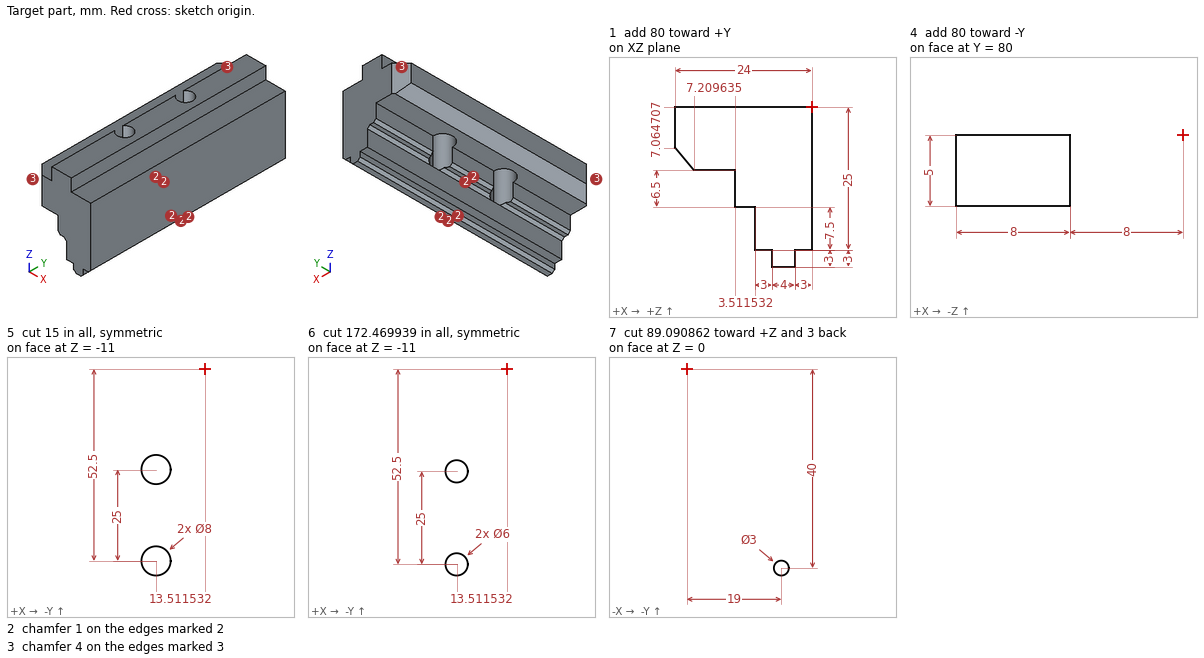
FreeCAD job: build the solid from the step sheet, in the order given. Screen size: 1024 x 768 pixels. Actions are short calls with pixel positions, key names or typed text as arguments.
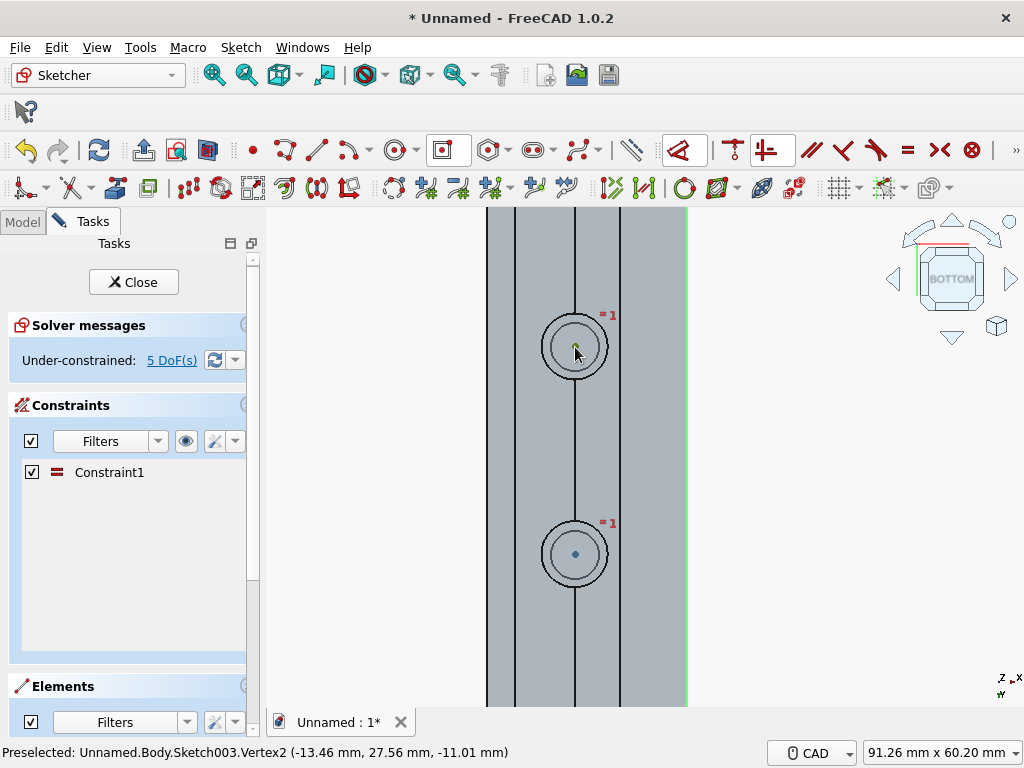
click(790, 150)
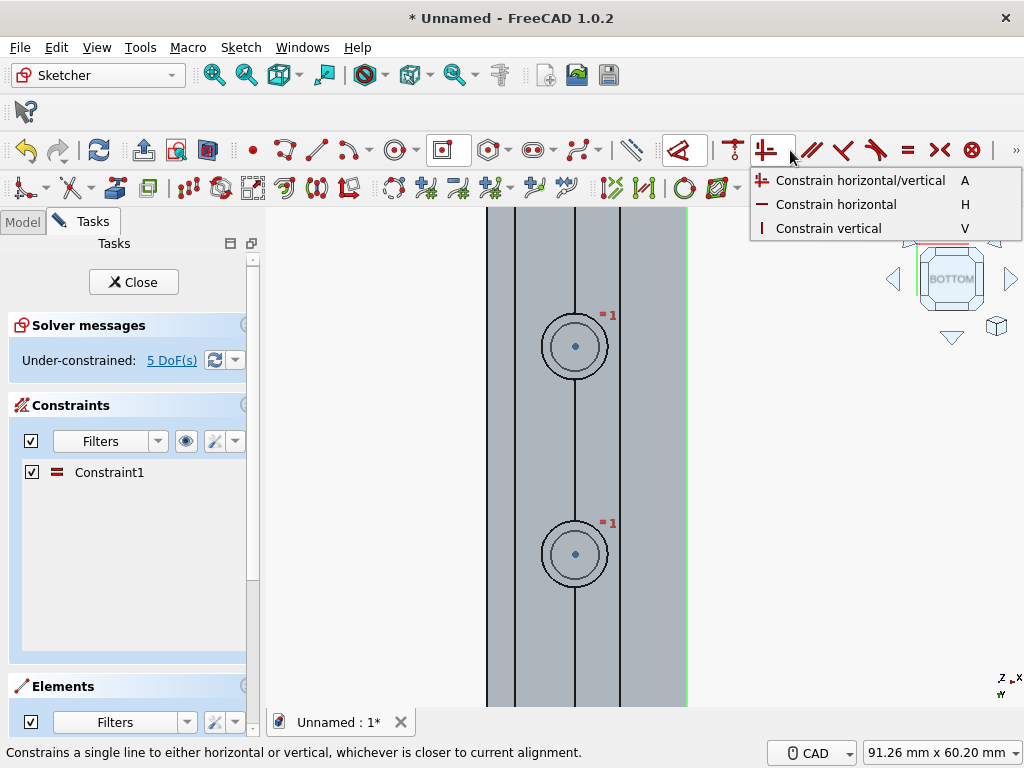
click(886, 228)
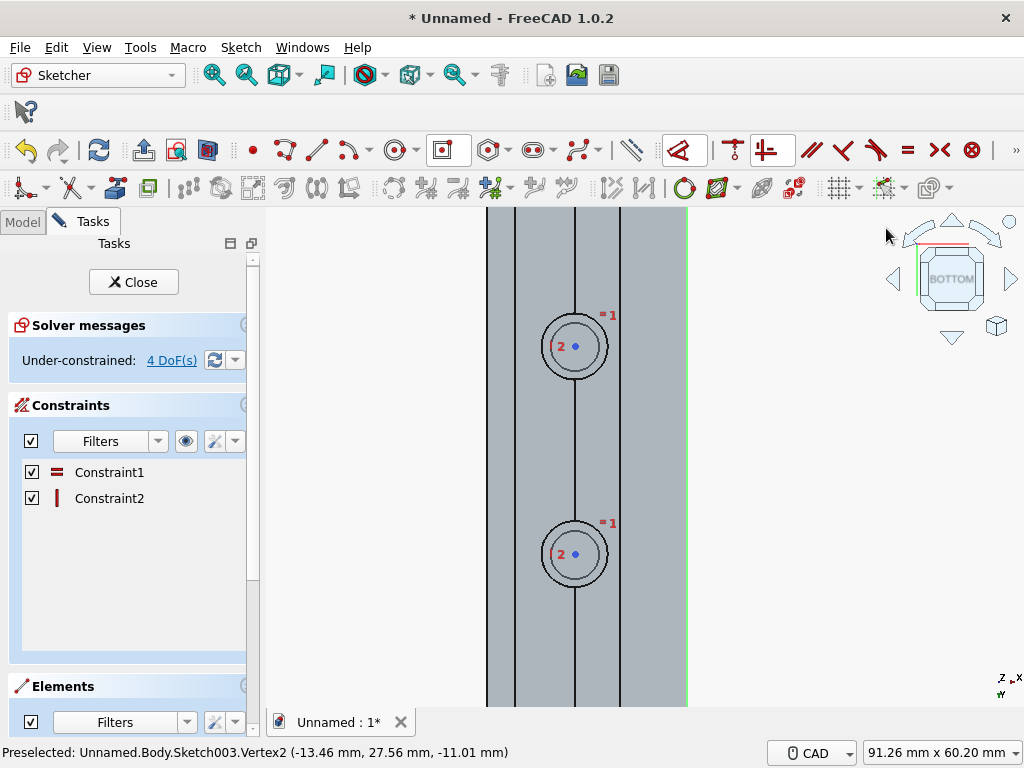
click(592, 538)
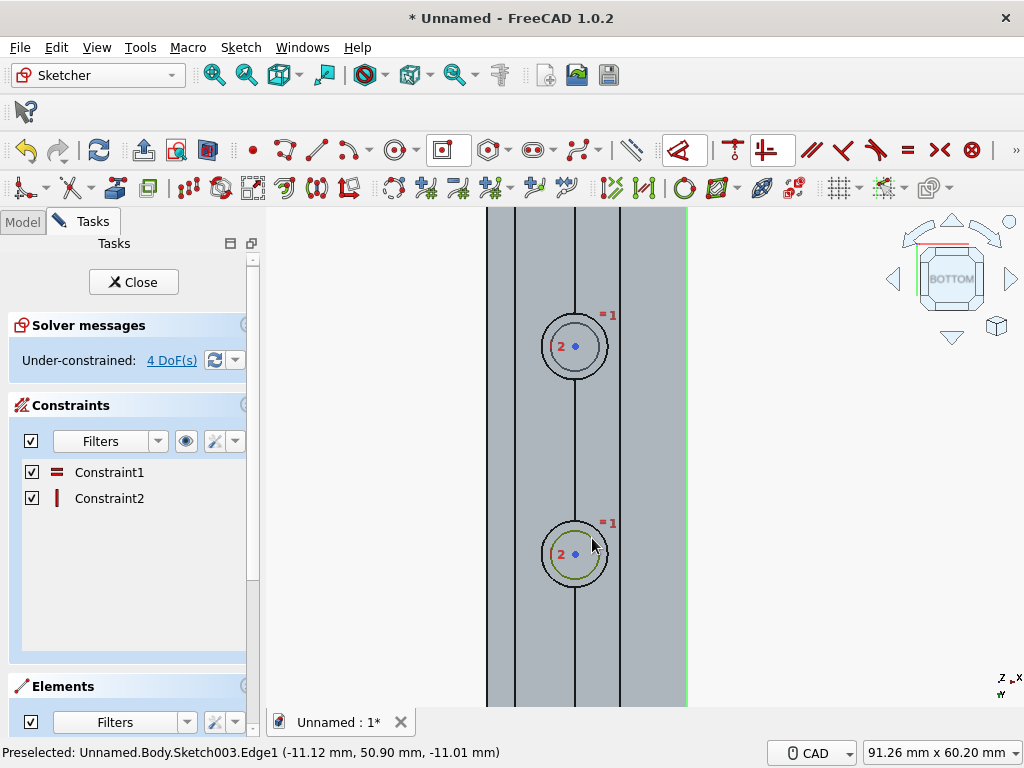
key(k)
key(o)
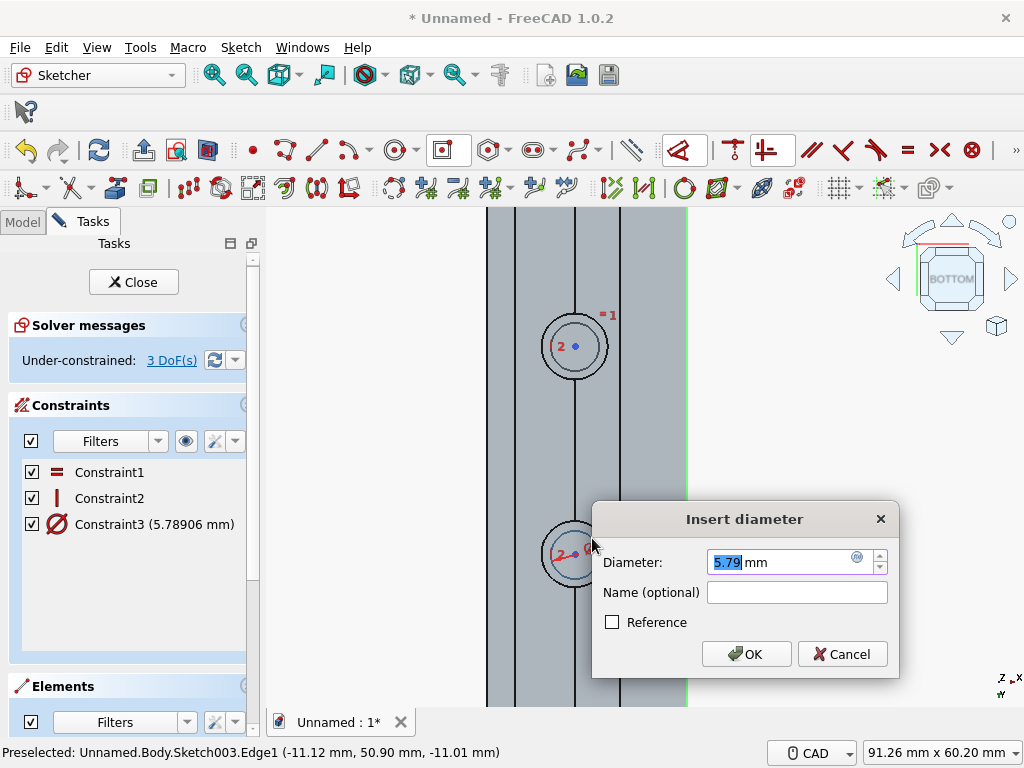
text(6)
key(Return)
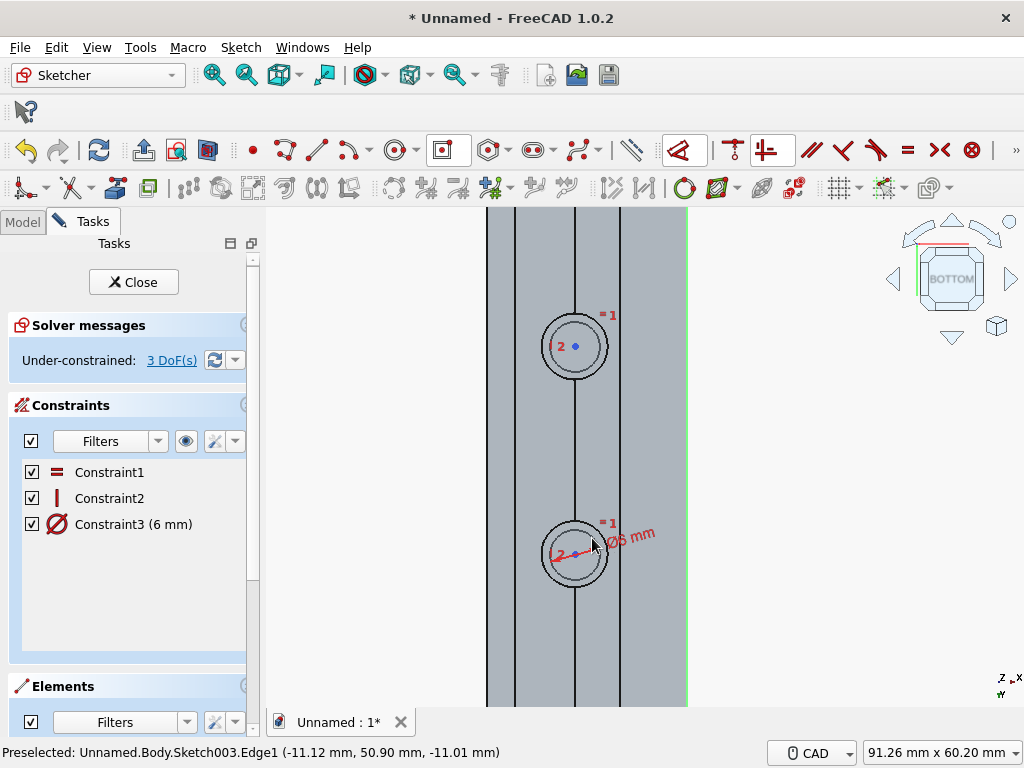
click(575, 555)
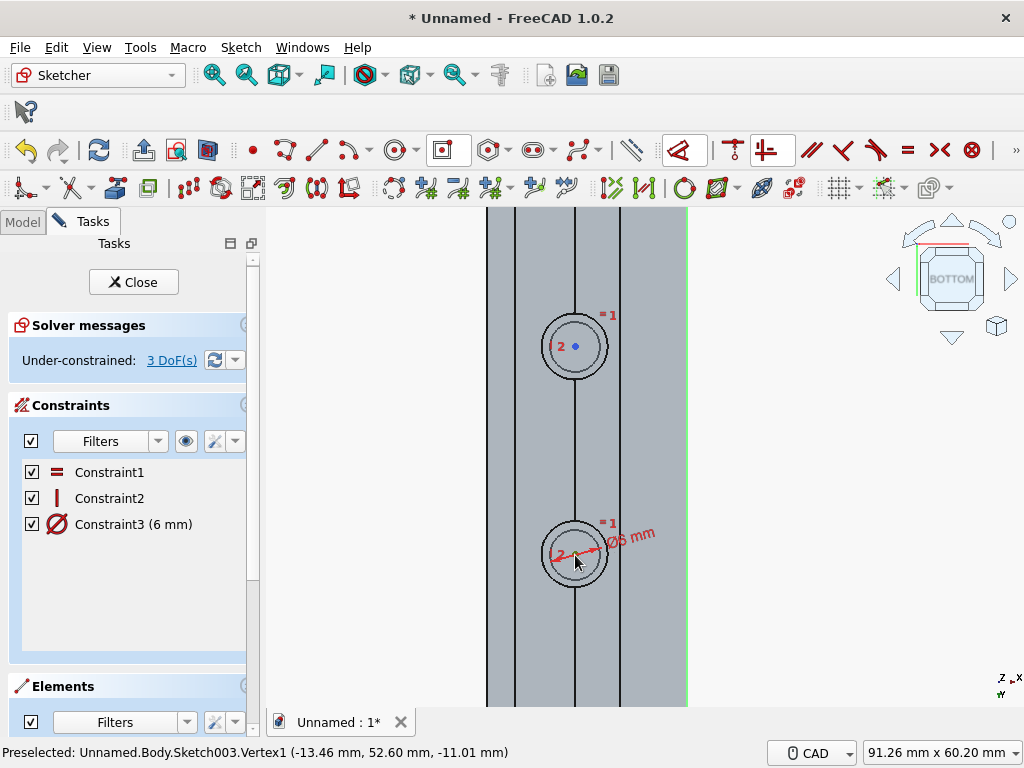
click(575, 347)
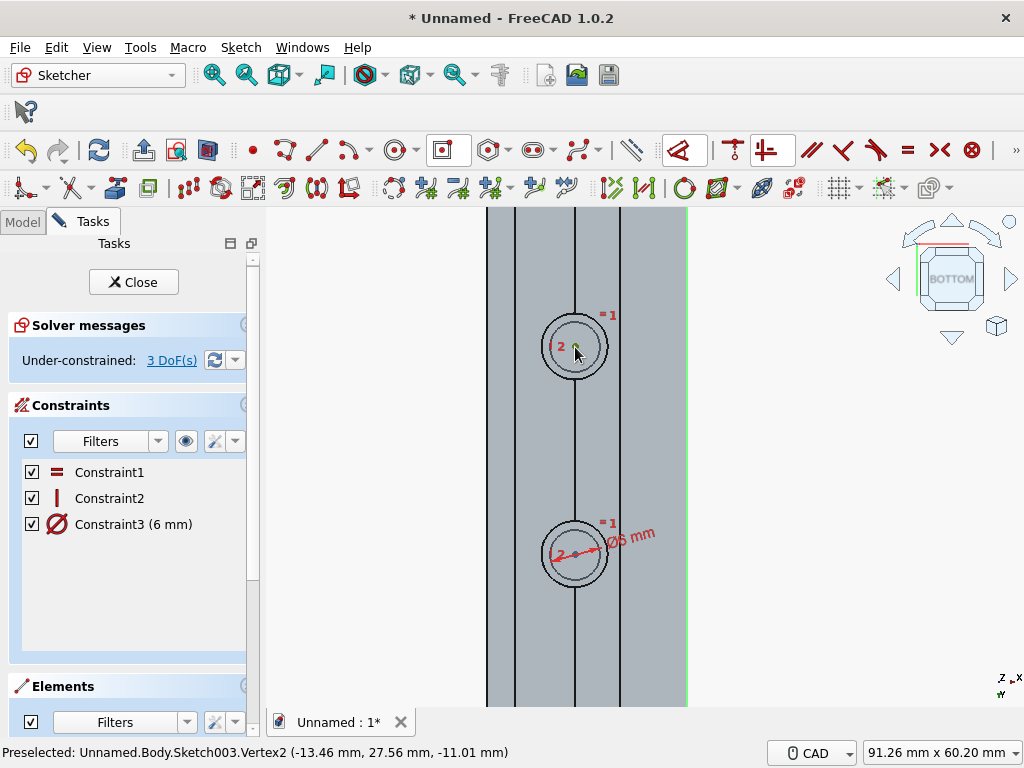
key(i)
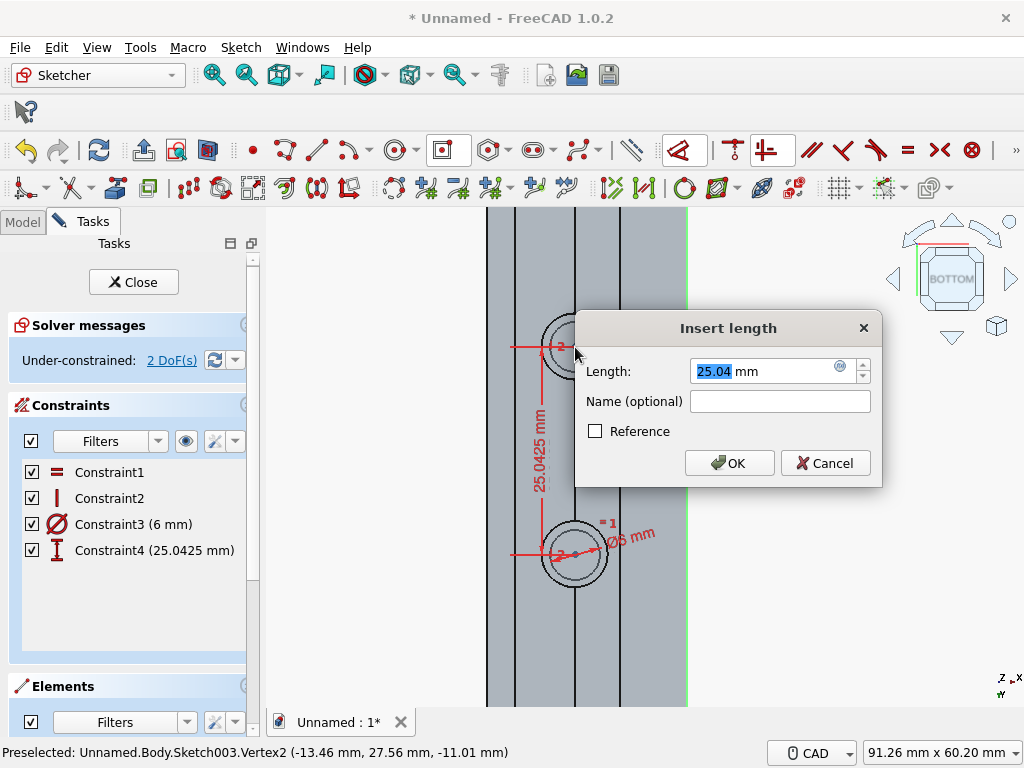
text(25)
key(Return)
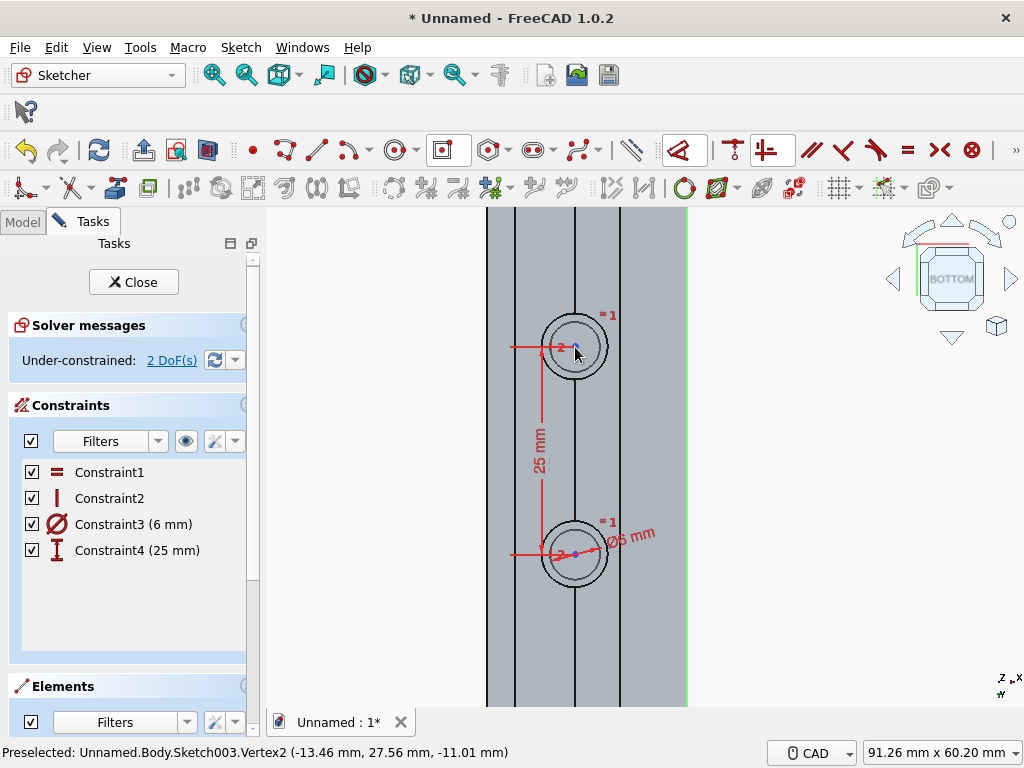
click(575, 555)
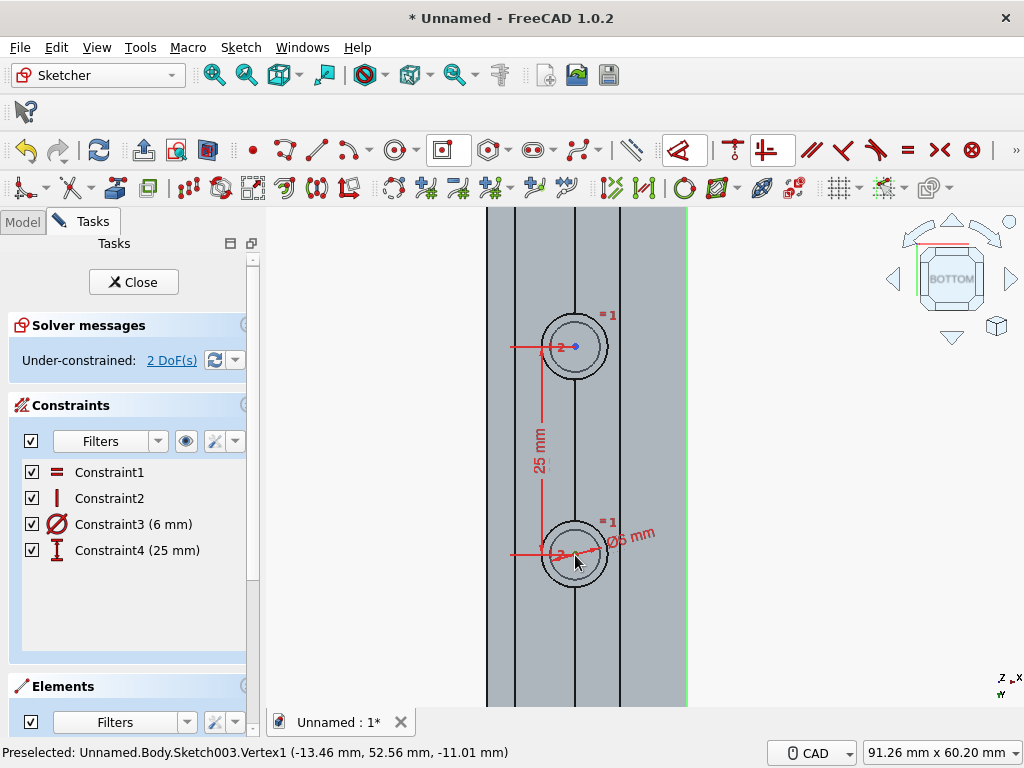
key(i)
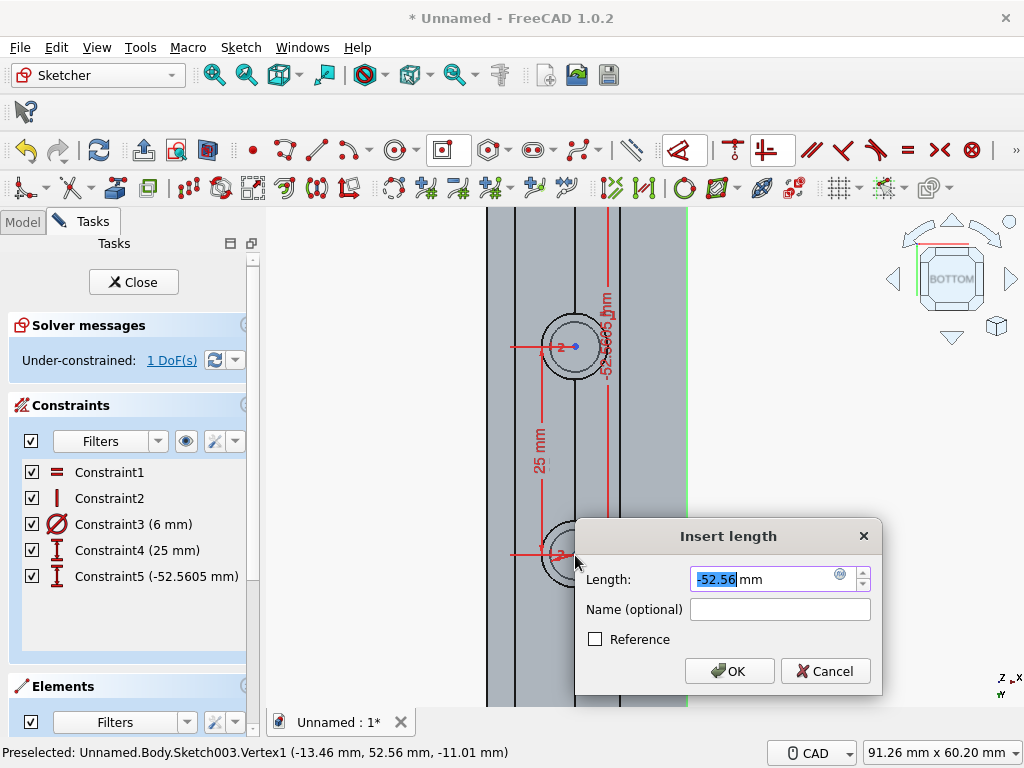
text(-52.5)
key(Return)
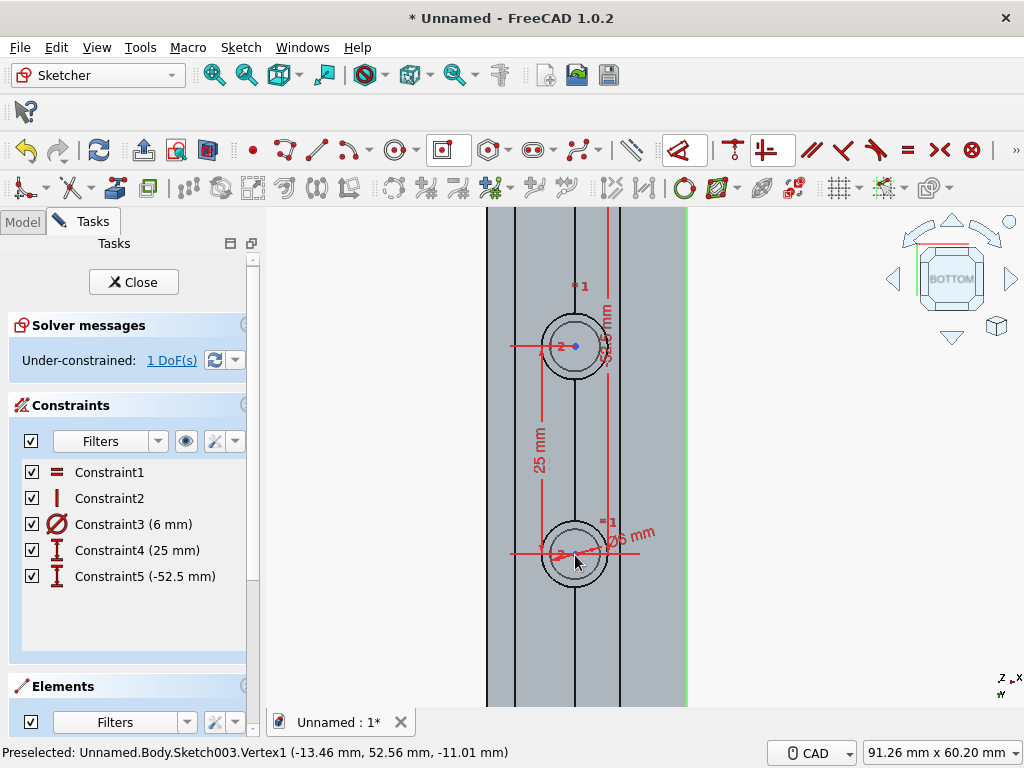
click(575, 554)